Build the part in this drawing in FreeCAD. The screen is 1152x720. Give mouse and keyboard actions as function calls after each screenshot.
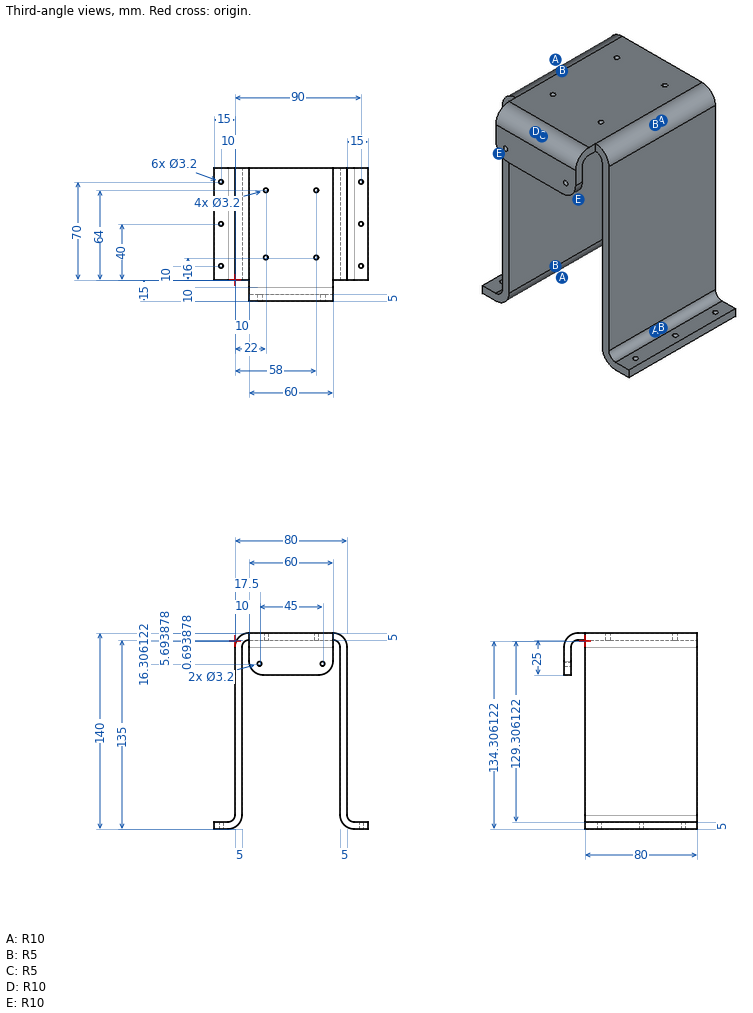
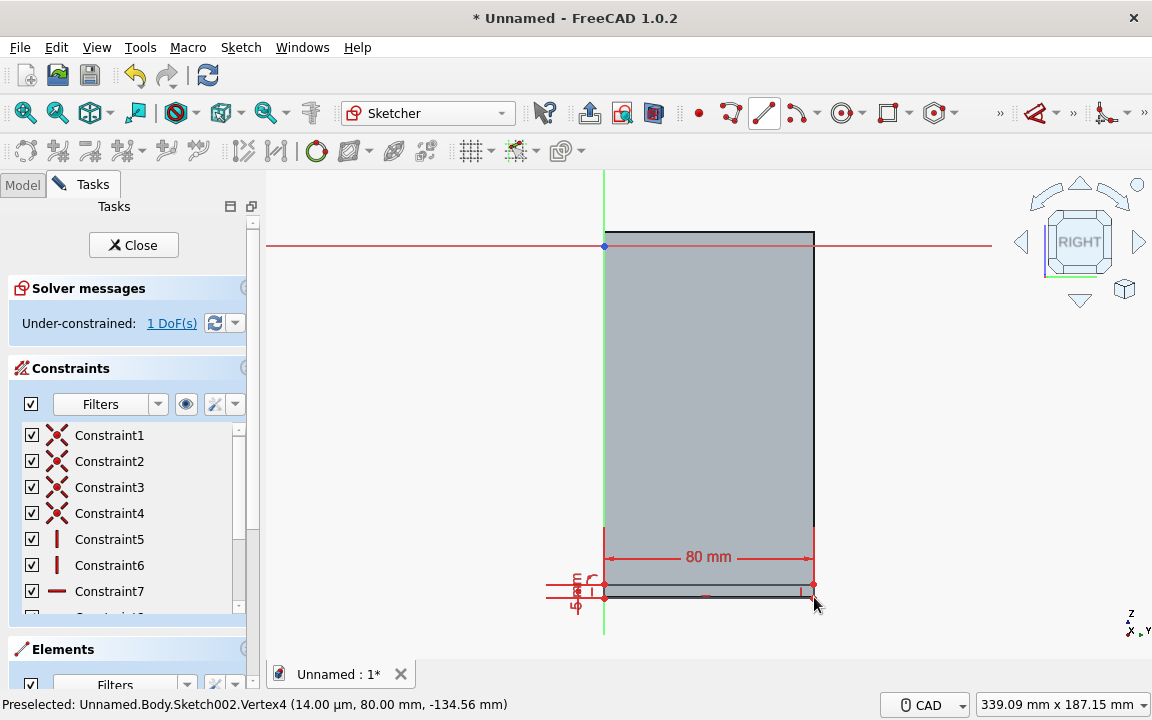
click(1036, 114)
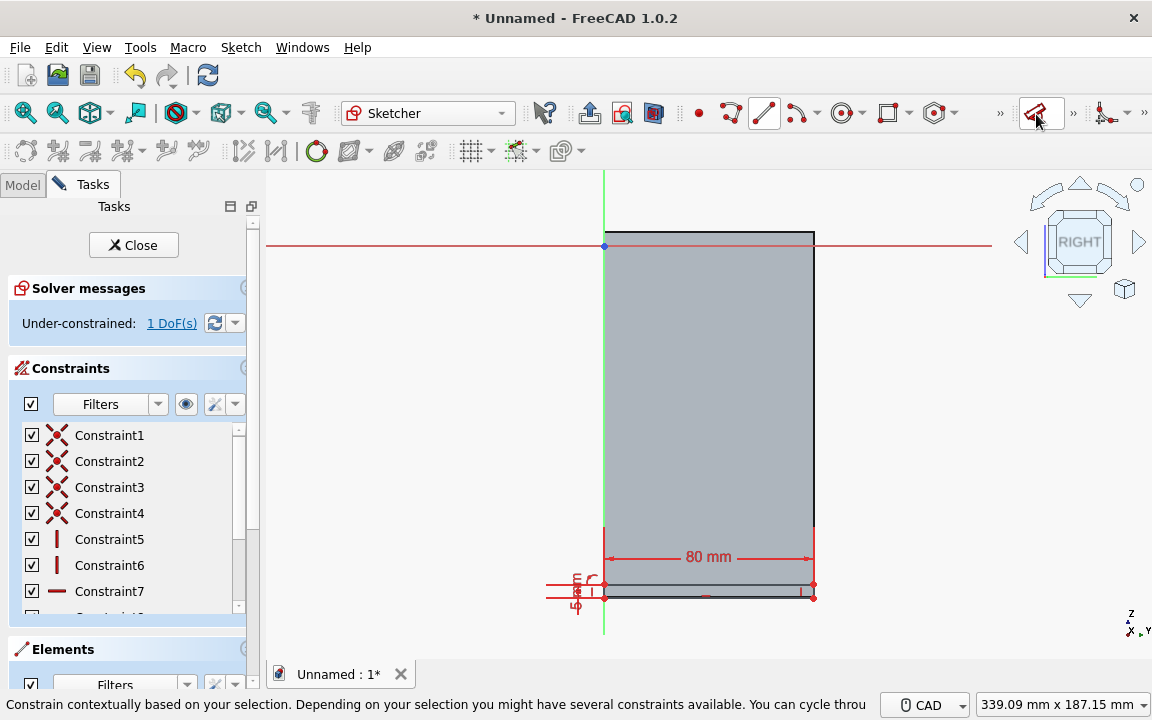
click(604, 585)
click(570, 416)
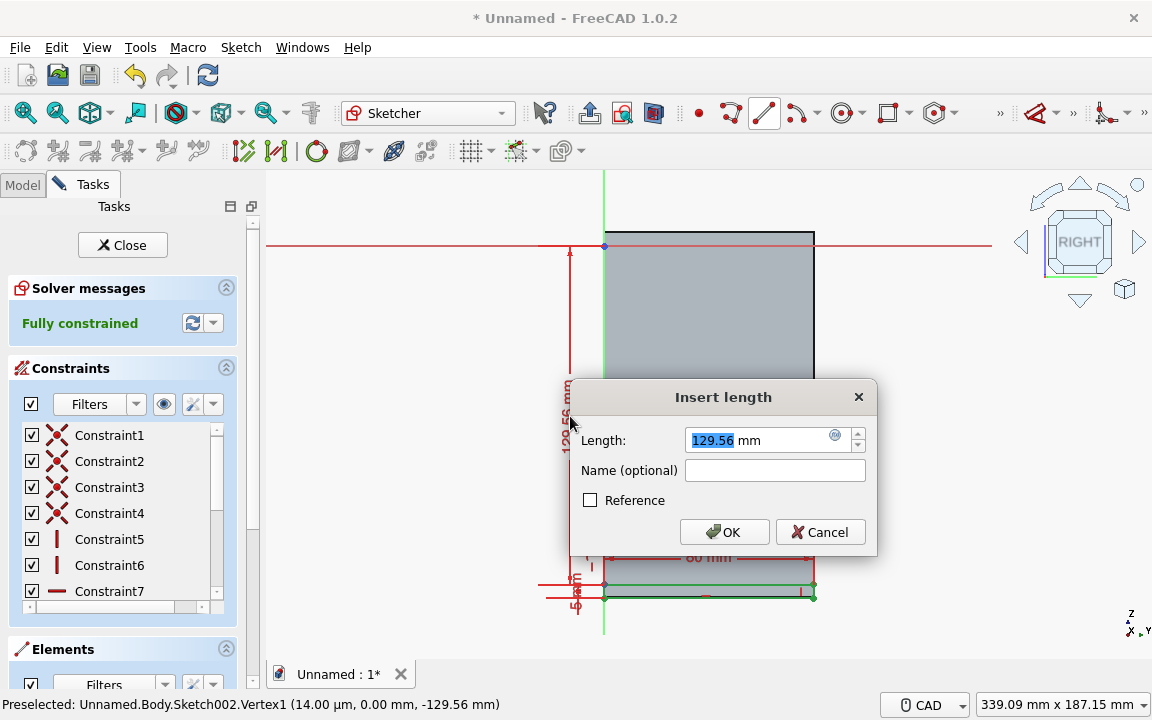
text(129.306122)
key(Return)
key(Escape)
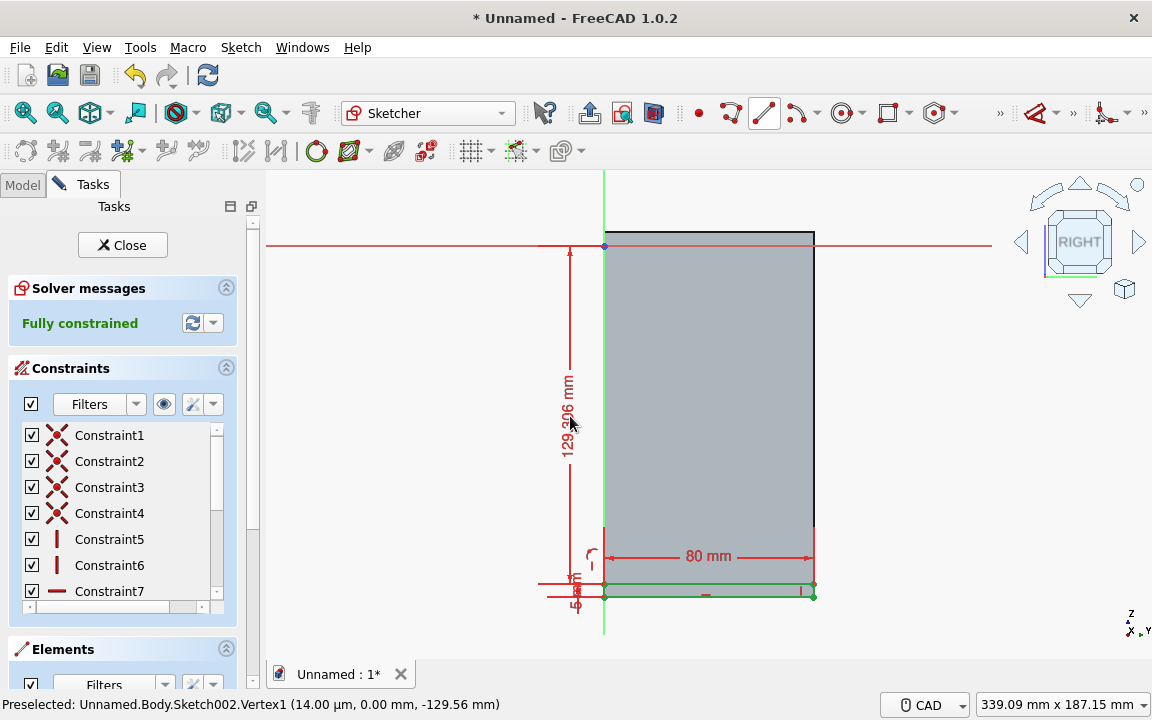
click(123, 245)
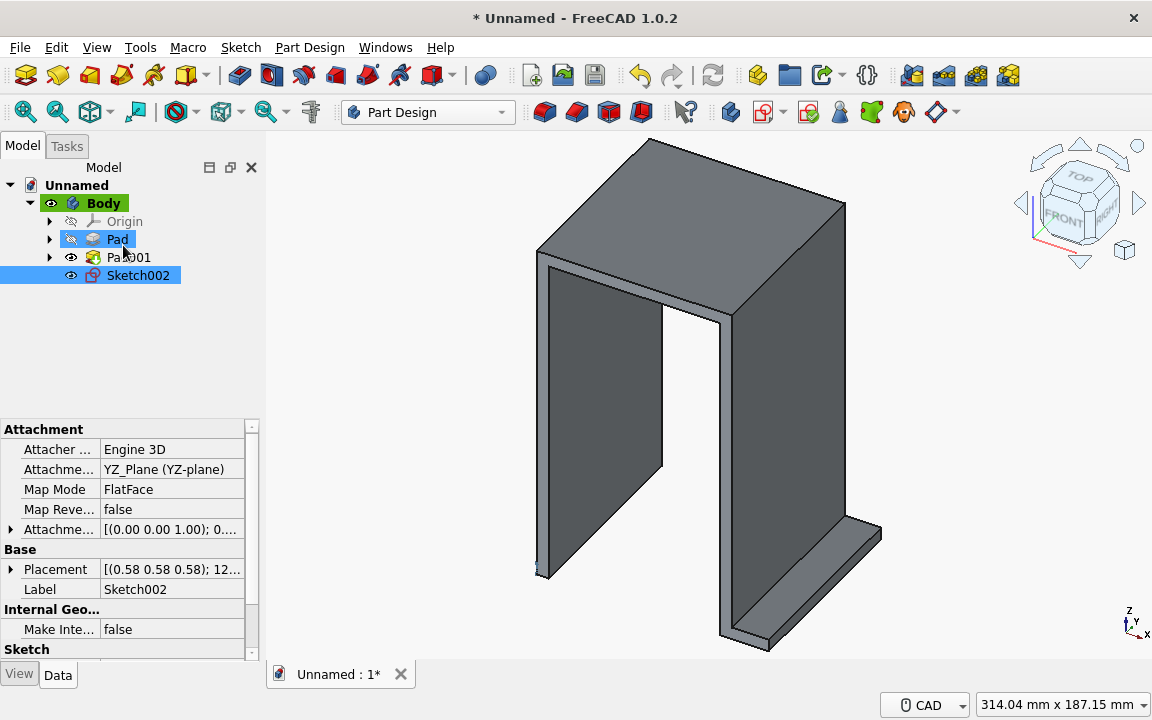
click(26, 76)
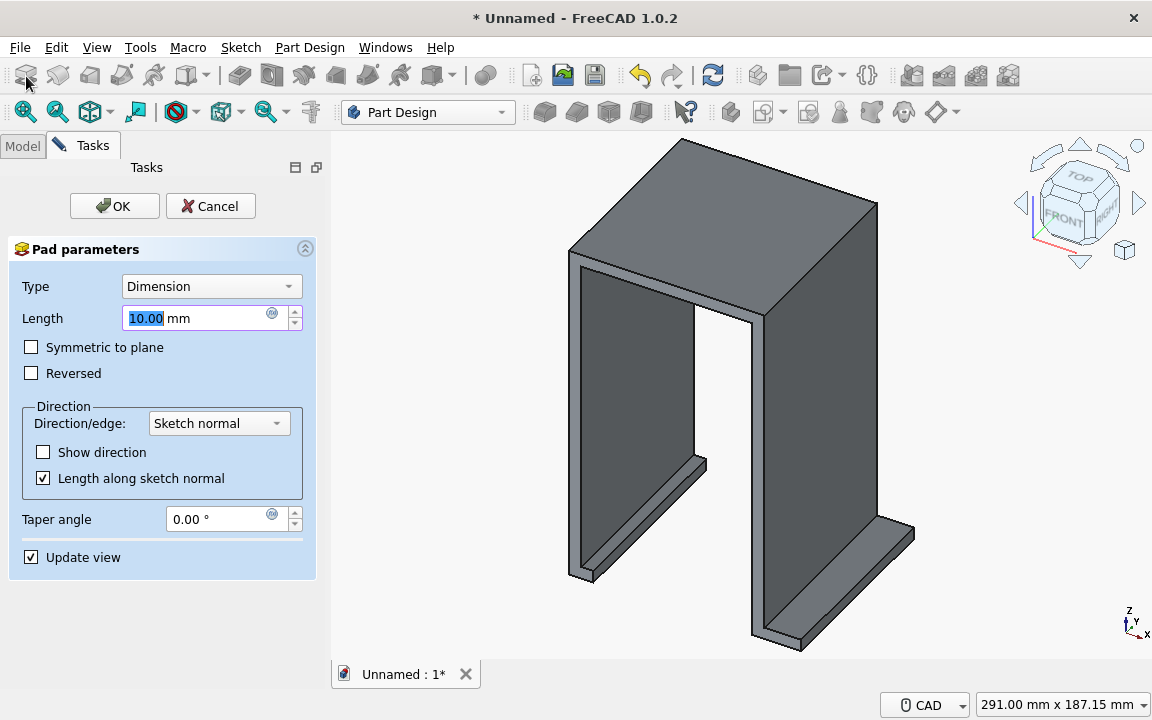
text(15)
key(Tab)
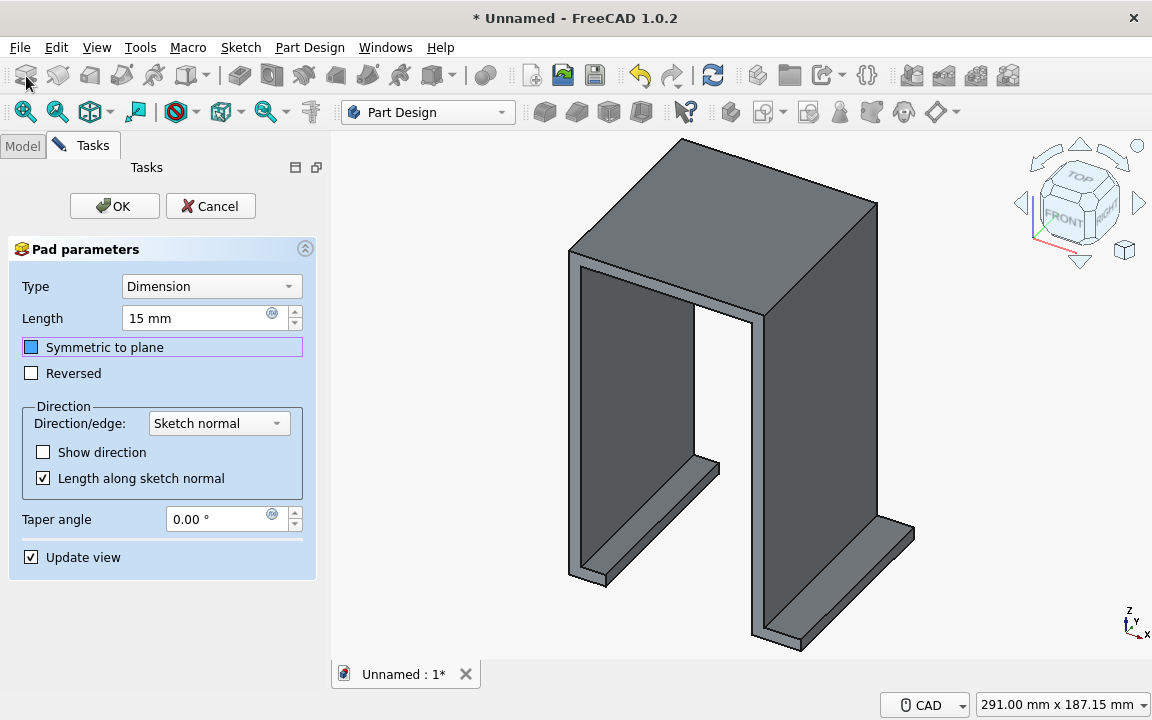
click(30, 373)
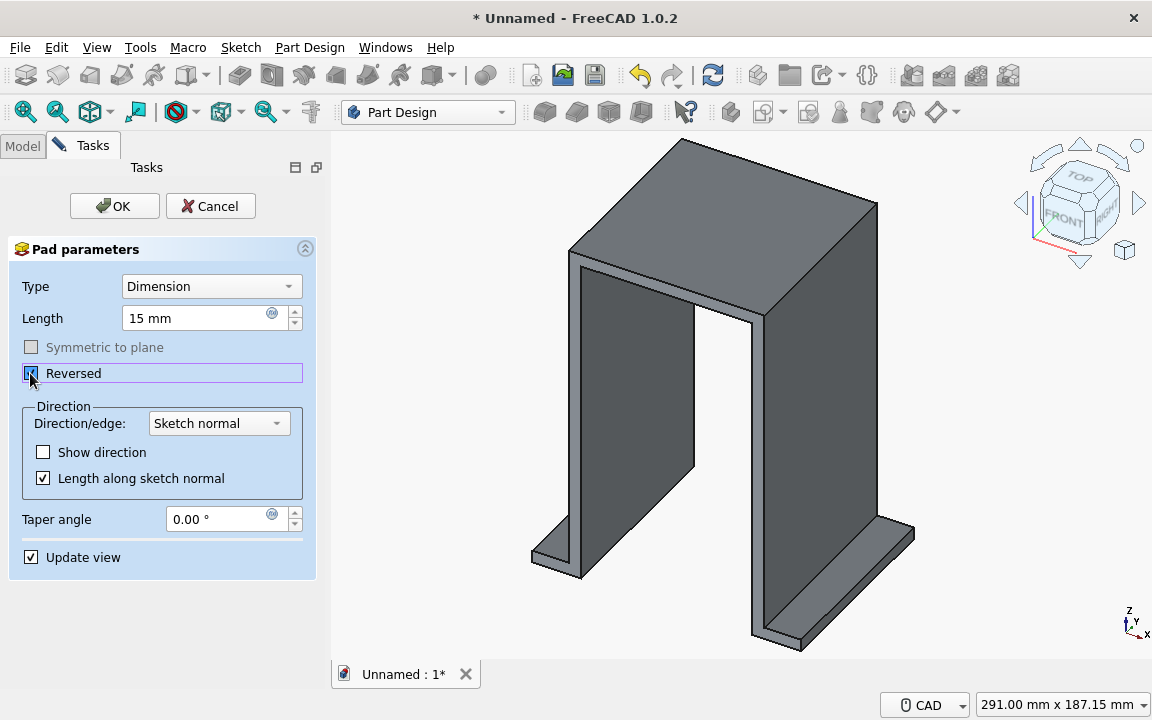
click(115, 206)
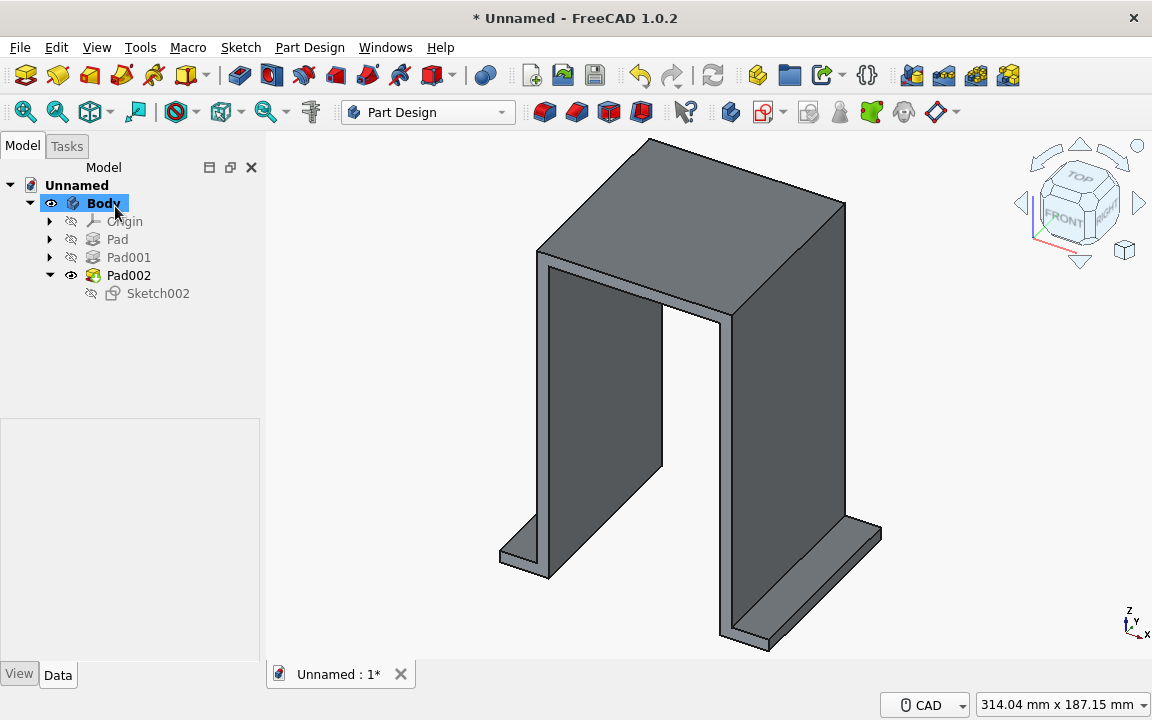
click(26, 112)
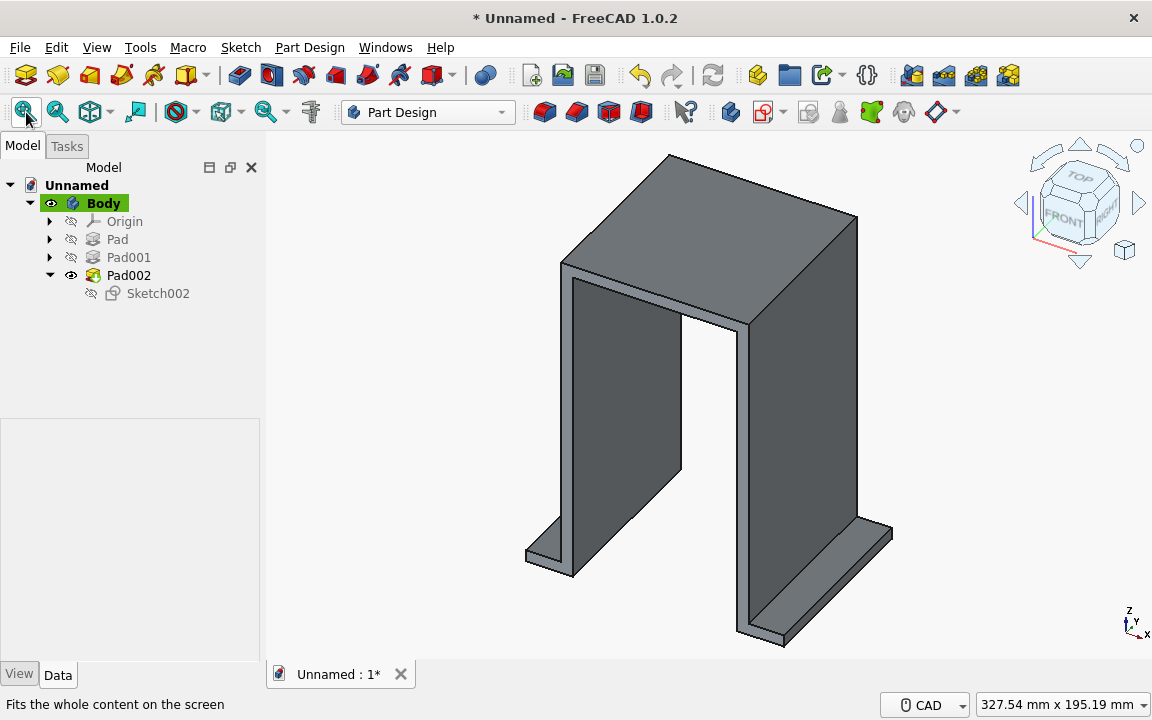
click(803, 270)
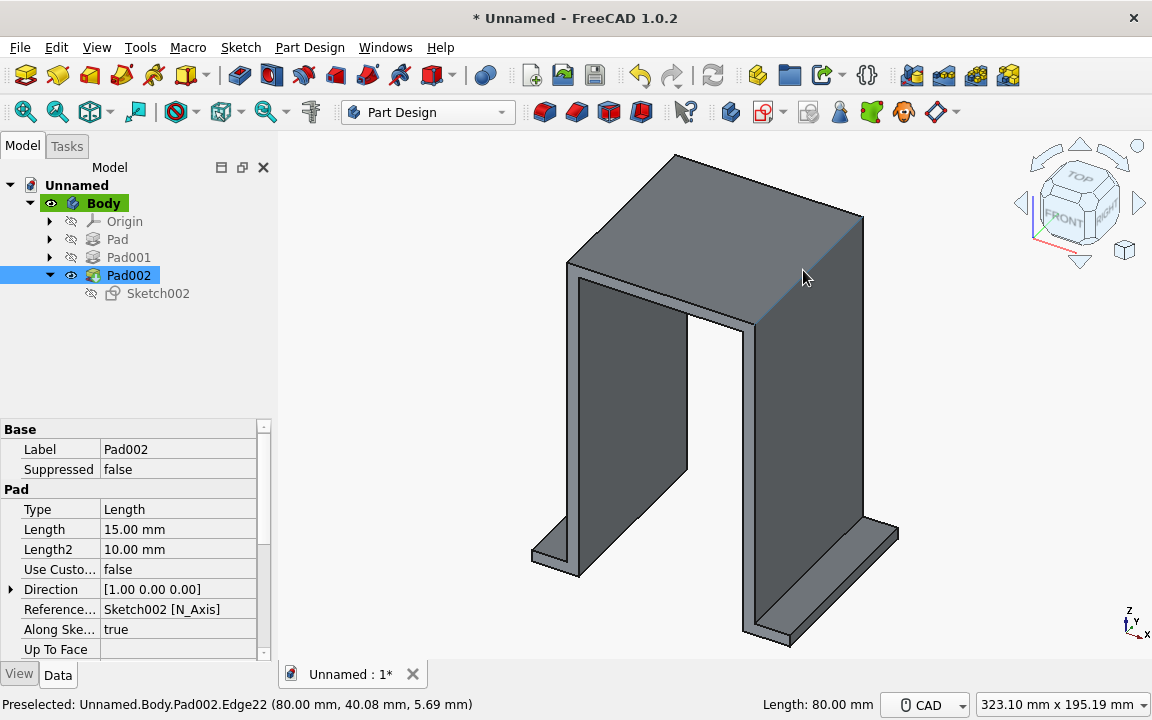
key(0)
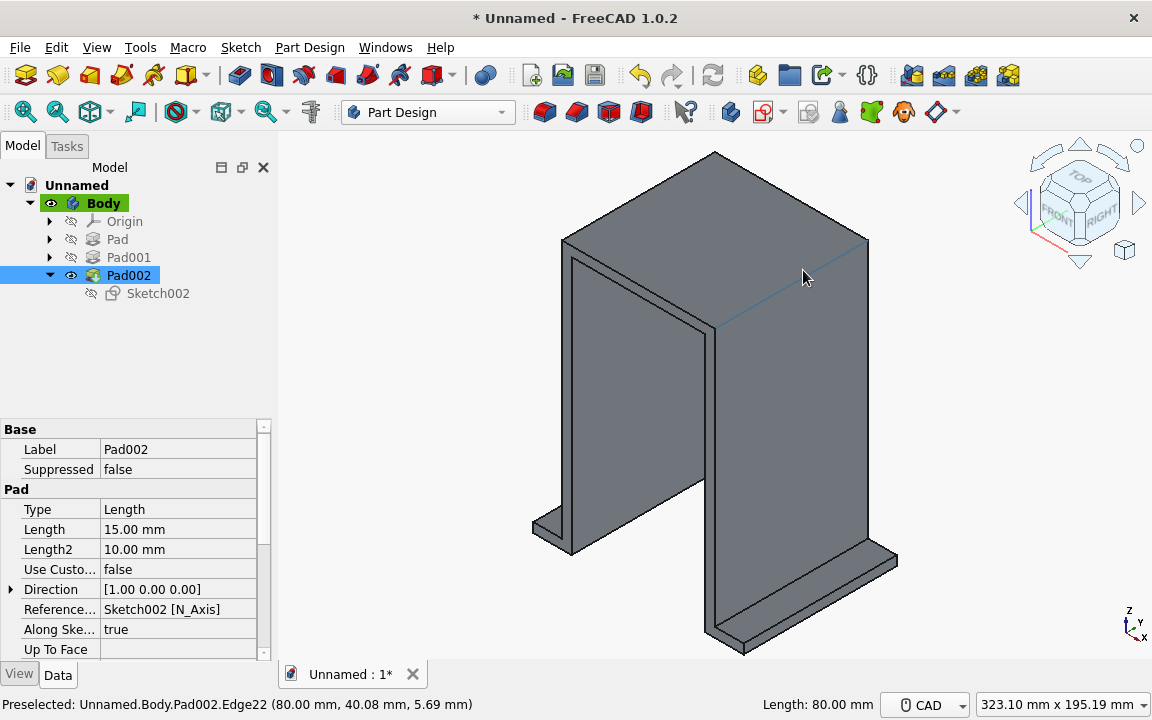
key(2)